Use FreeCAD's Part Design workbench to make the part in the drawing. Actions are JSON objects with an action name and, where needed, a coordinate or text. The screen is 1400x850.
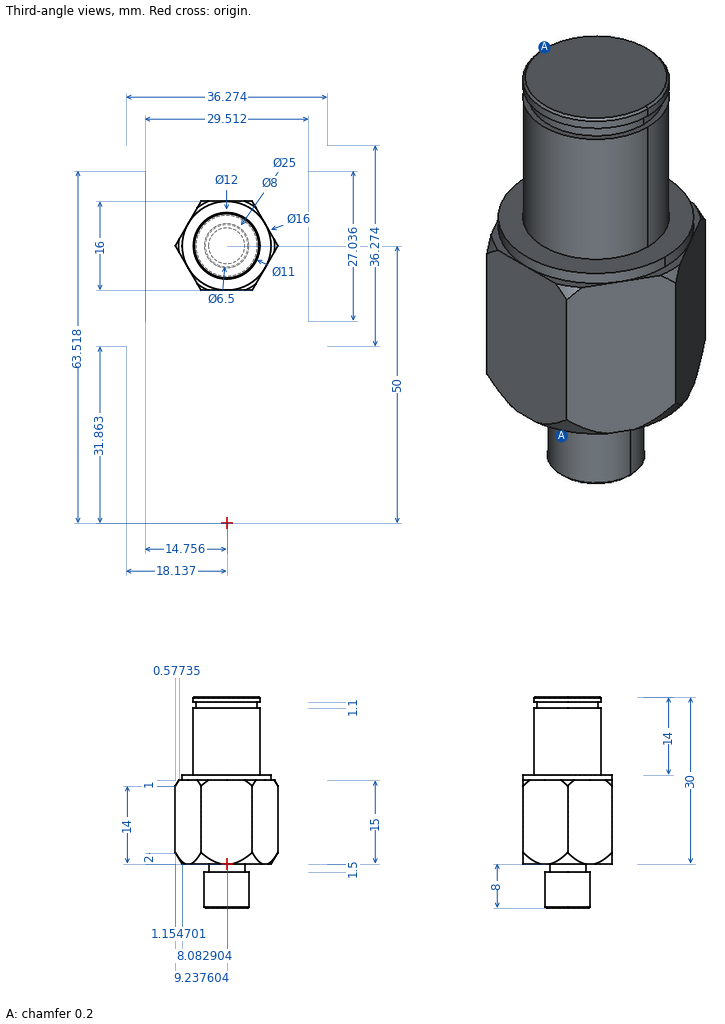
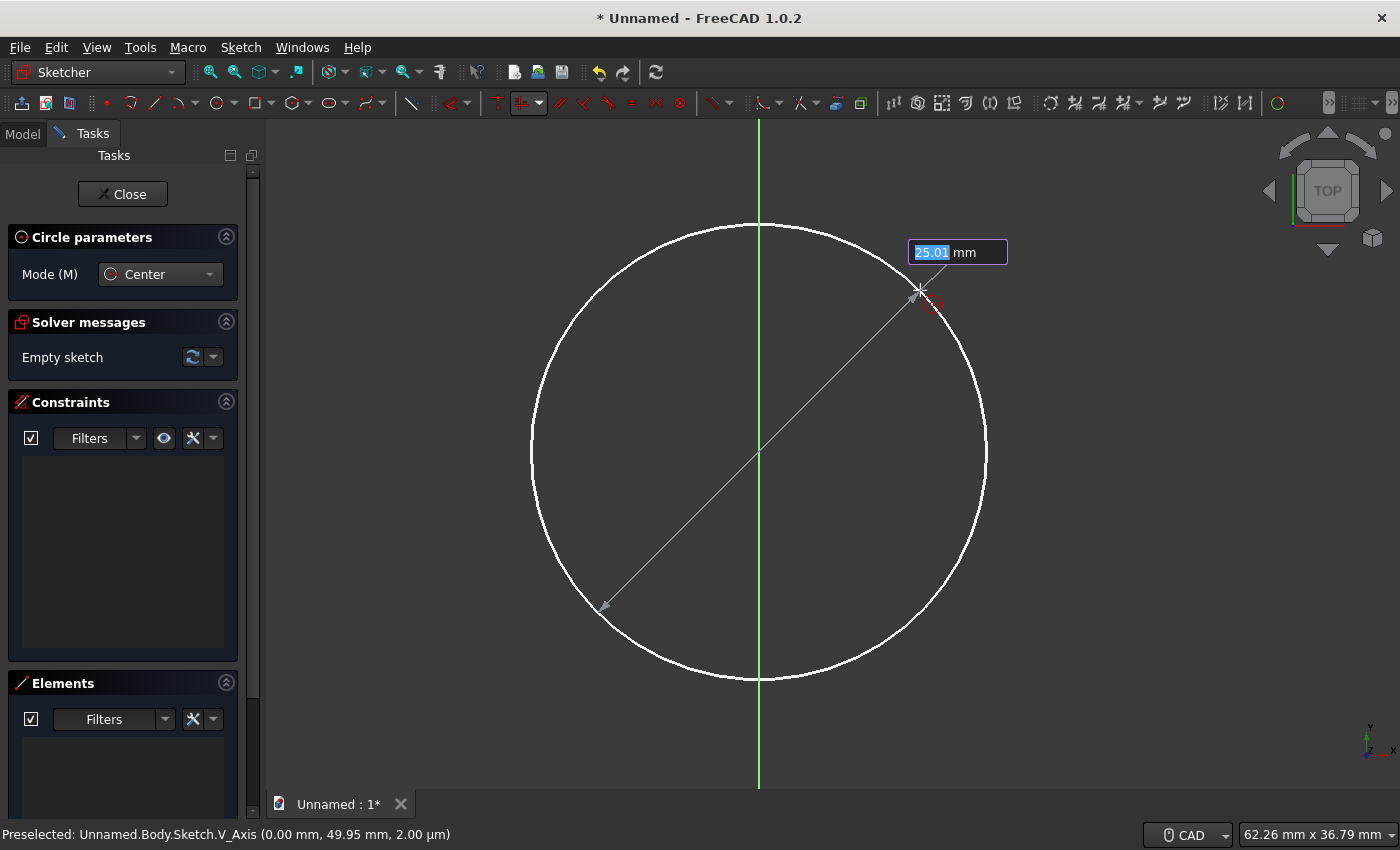
{"action": "type", "text": "25"}
{"action": "key", "text": "Return"}
{"action": "key", "text": "Escape"}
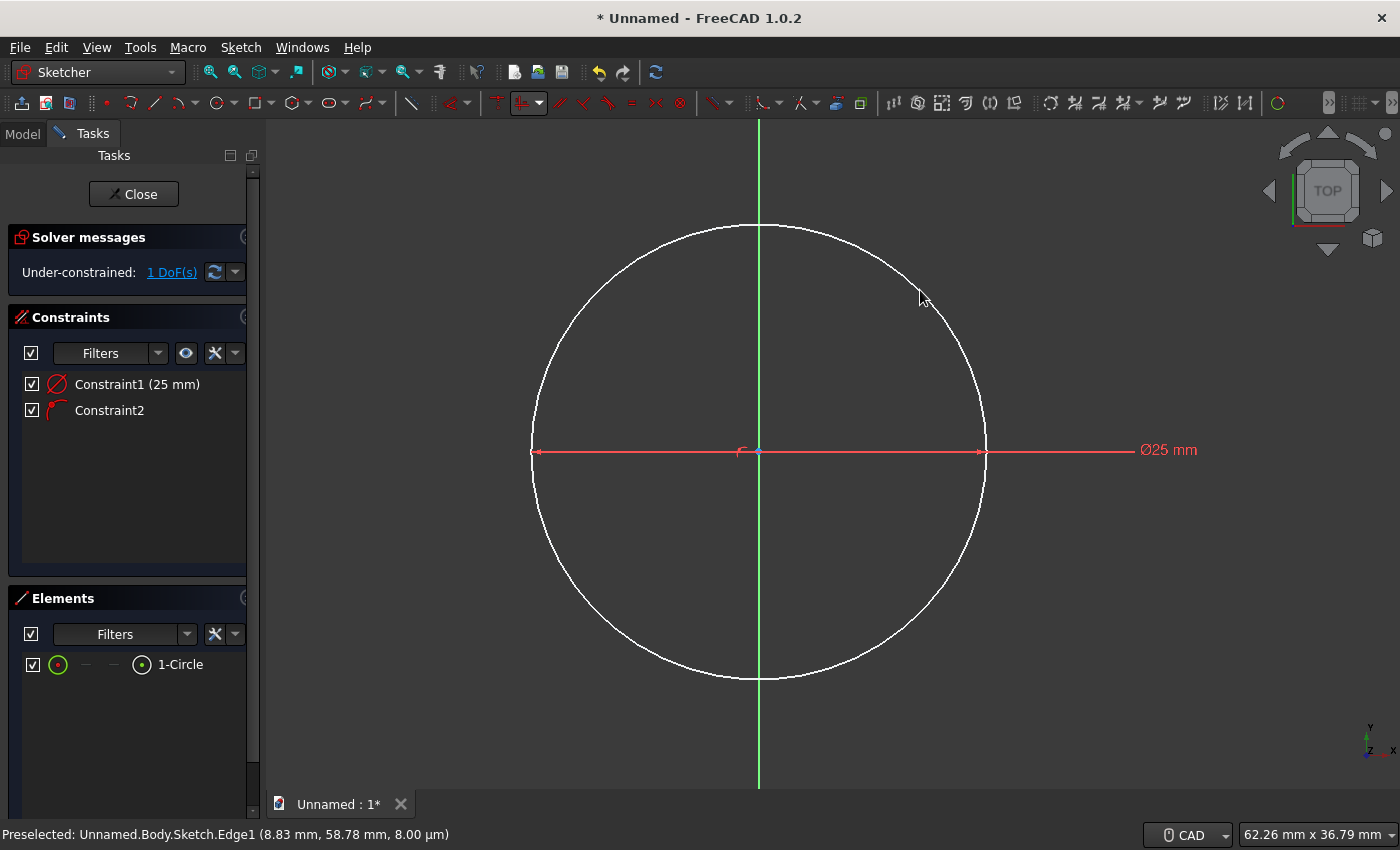
{"action": "left_click", "coordinate": [450, 104]}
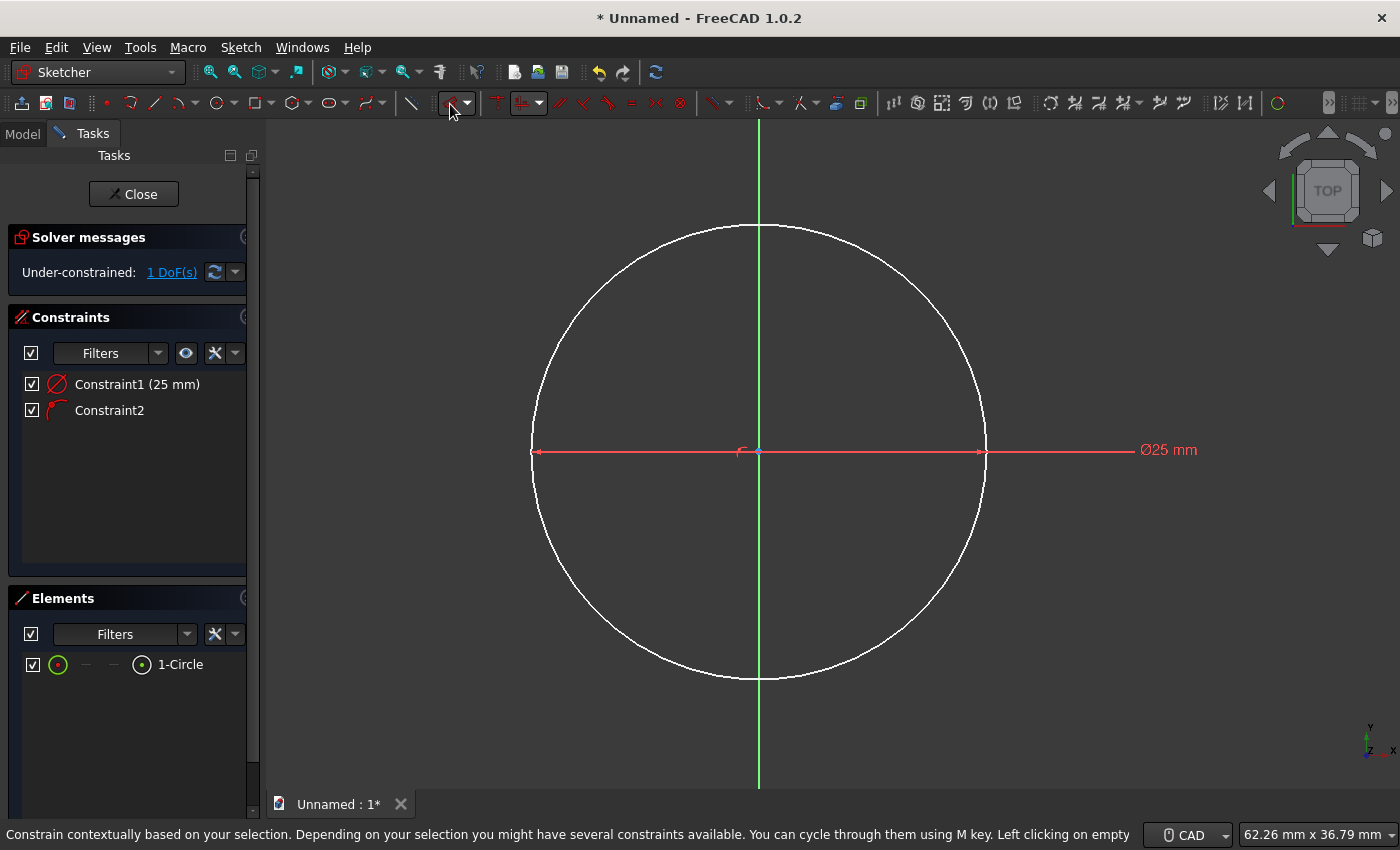
{"action": "left_click", "coordinate": [759, 452]}
{"action": "left_click", "coordinate": [793, 607]}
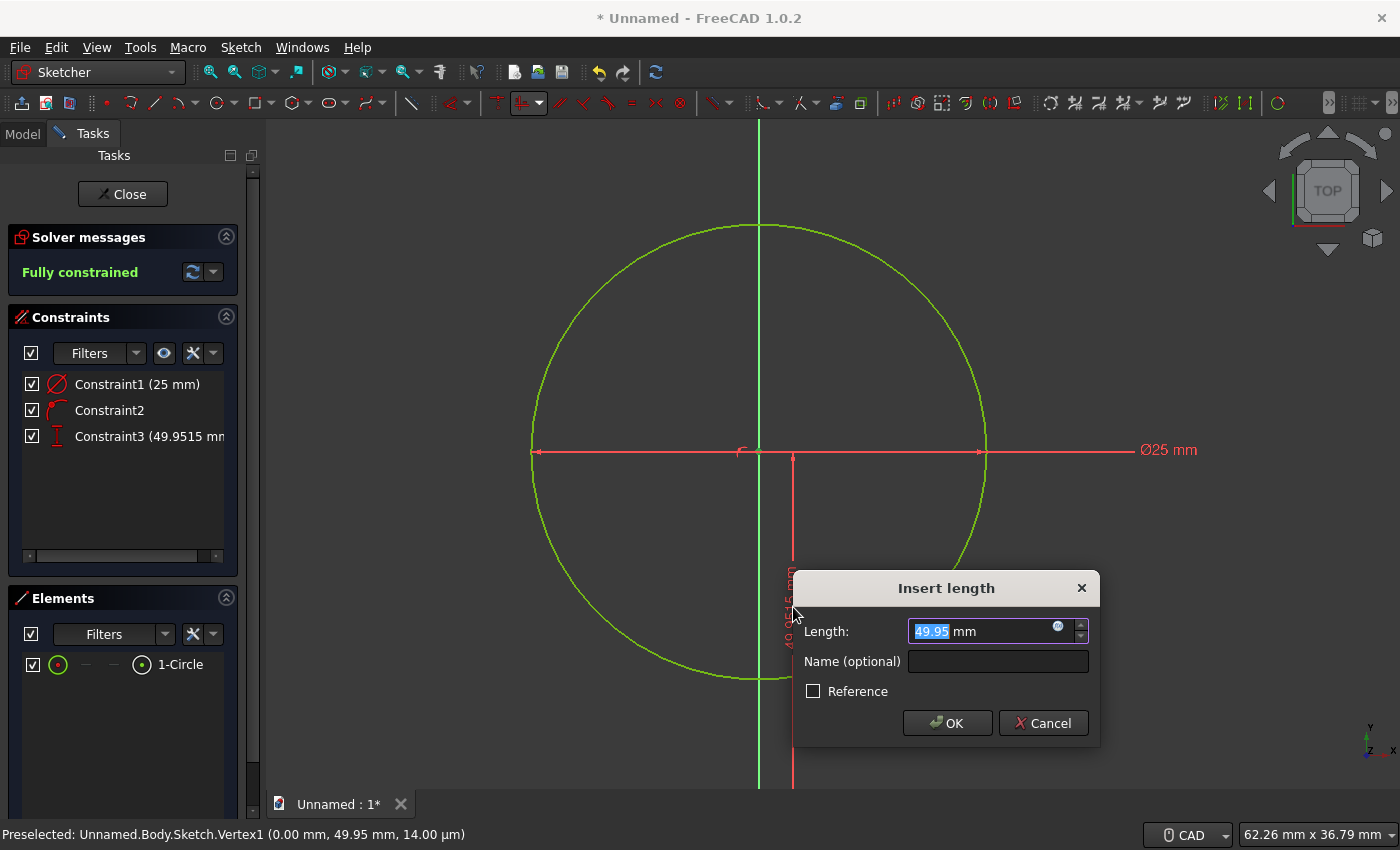
{"action": "type", "text": "50"}
{"action": "key", "text": "Return"}
{"action": "key", "text": "Escape"}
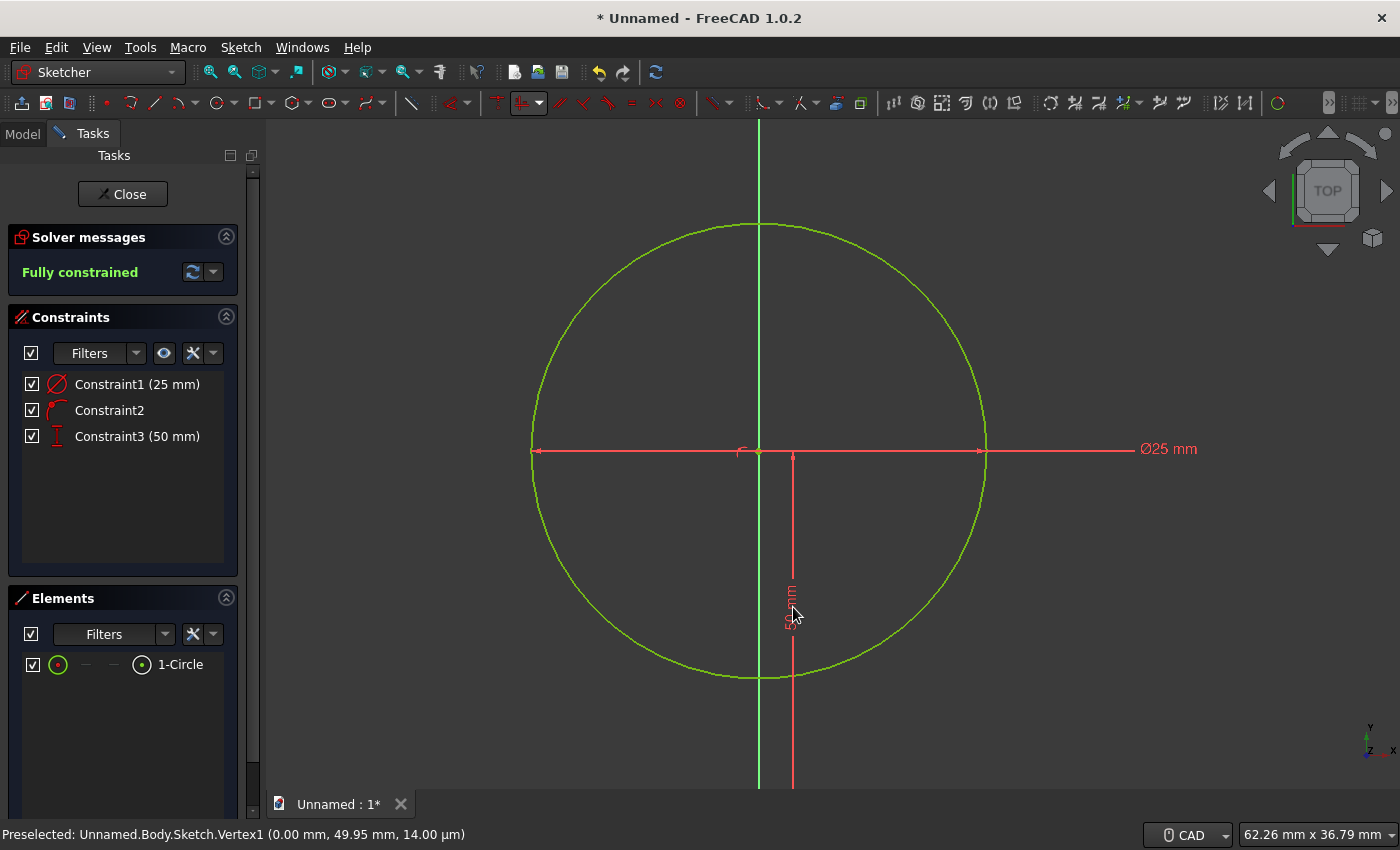
{"action": "left_click", "coordinate": [123, 194]}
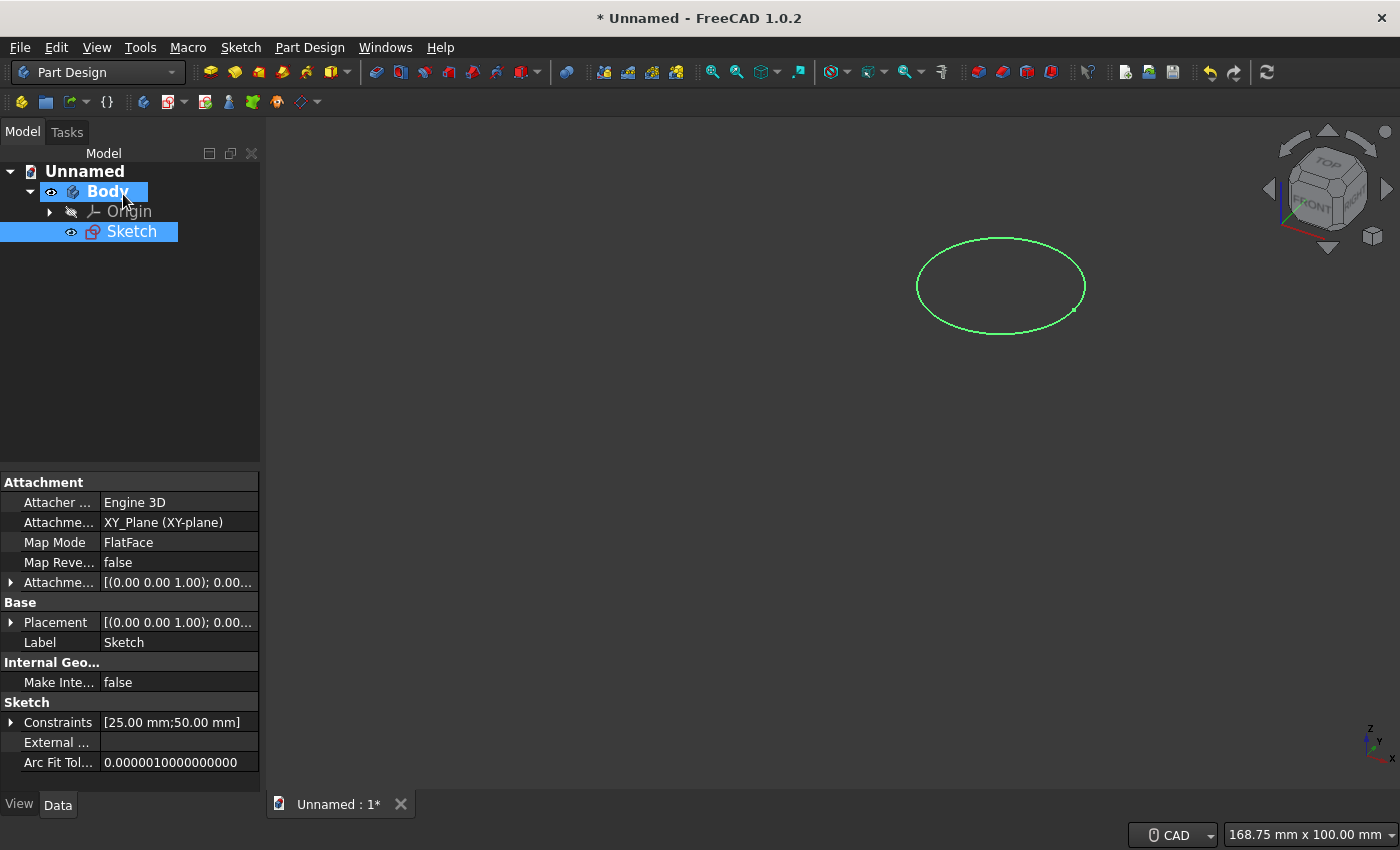
{"action": "left_click", "coordinate": [212, 72]}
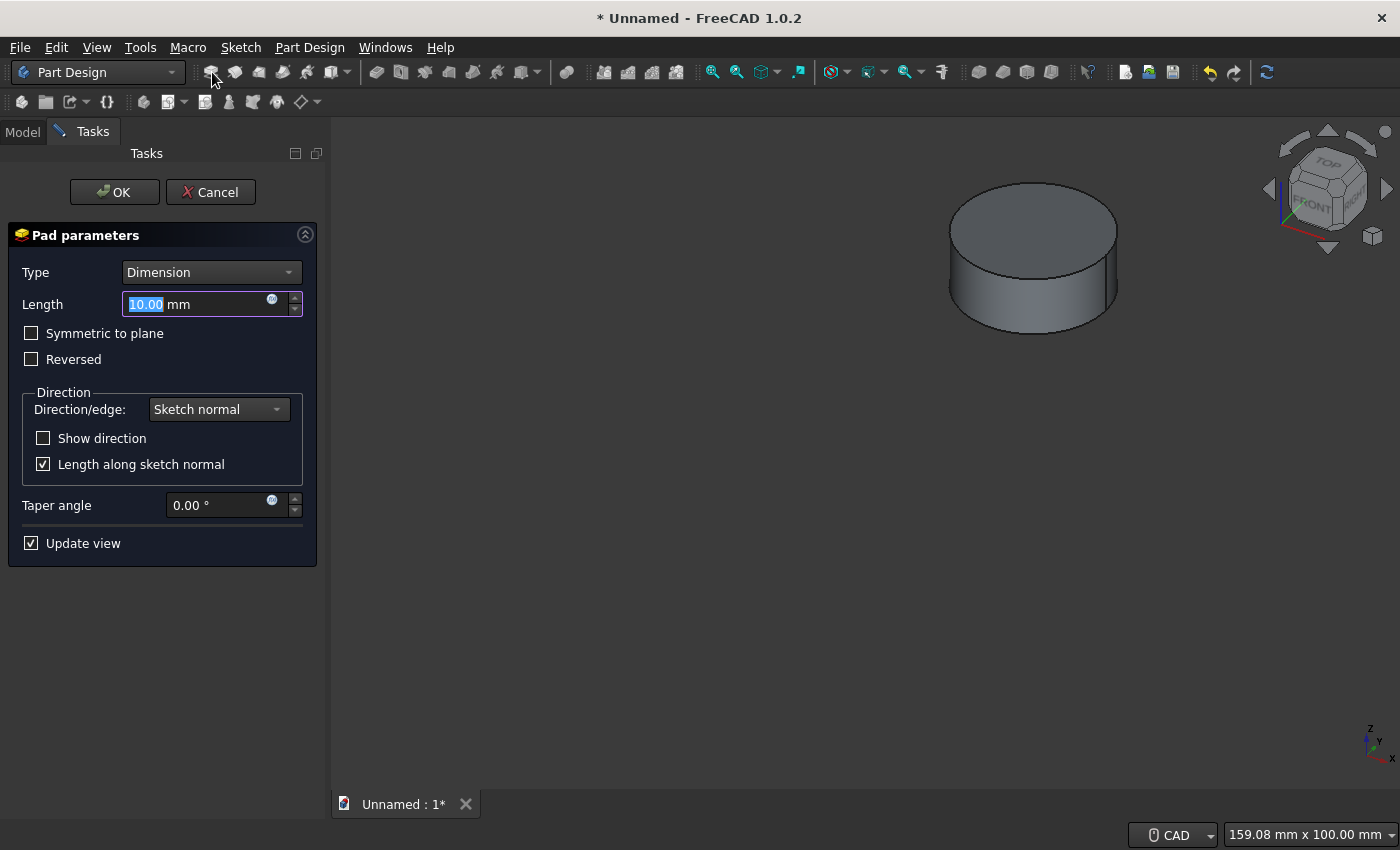
{"action": "type", "text": "30"}
{"action": "key", "text": "Tab"}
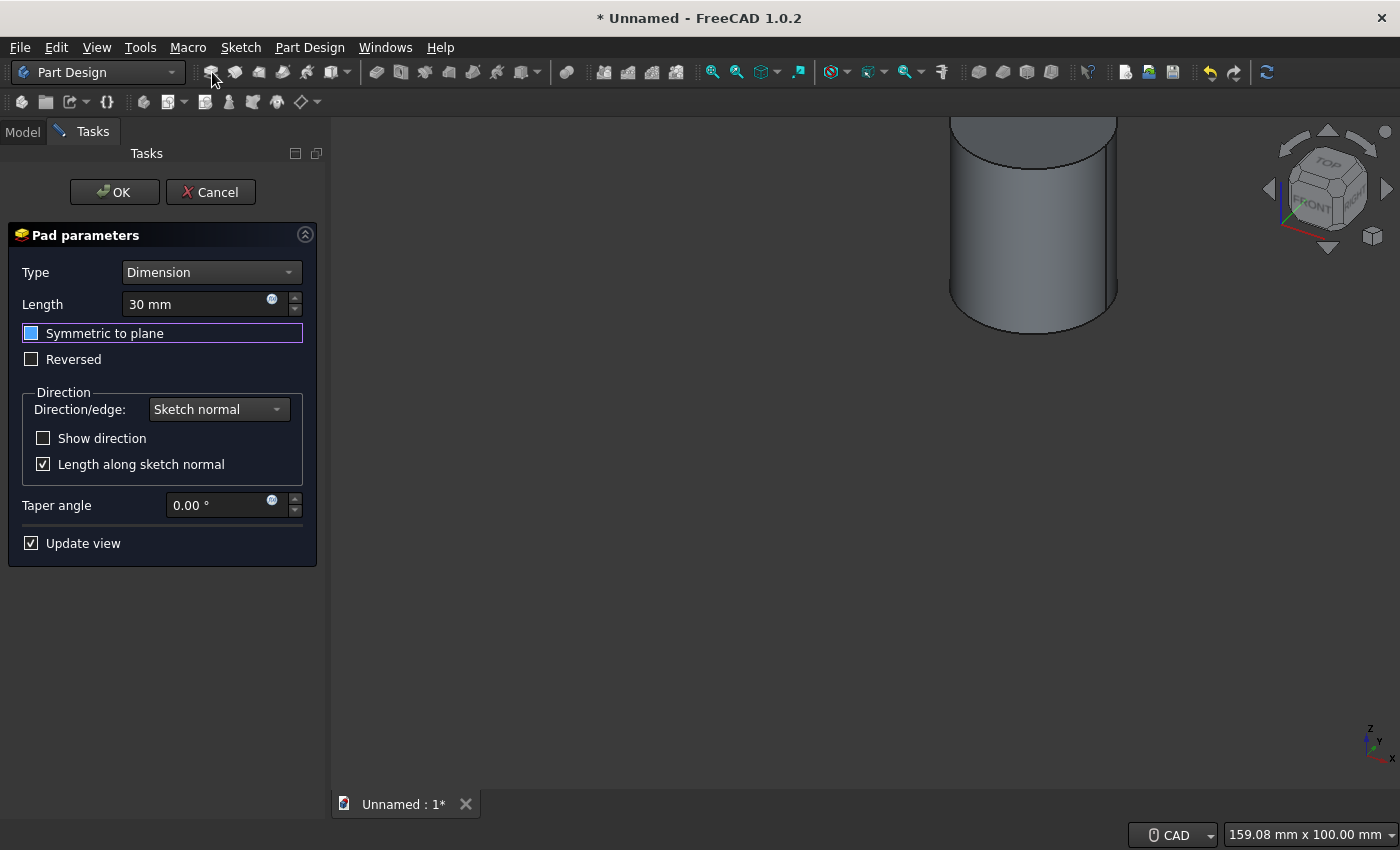
{"action": "left_click", "coordinate": [115, 192]}